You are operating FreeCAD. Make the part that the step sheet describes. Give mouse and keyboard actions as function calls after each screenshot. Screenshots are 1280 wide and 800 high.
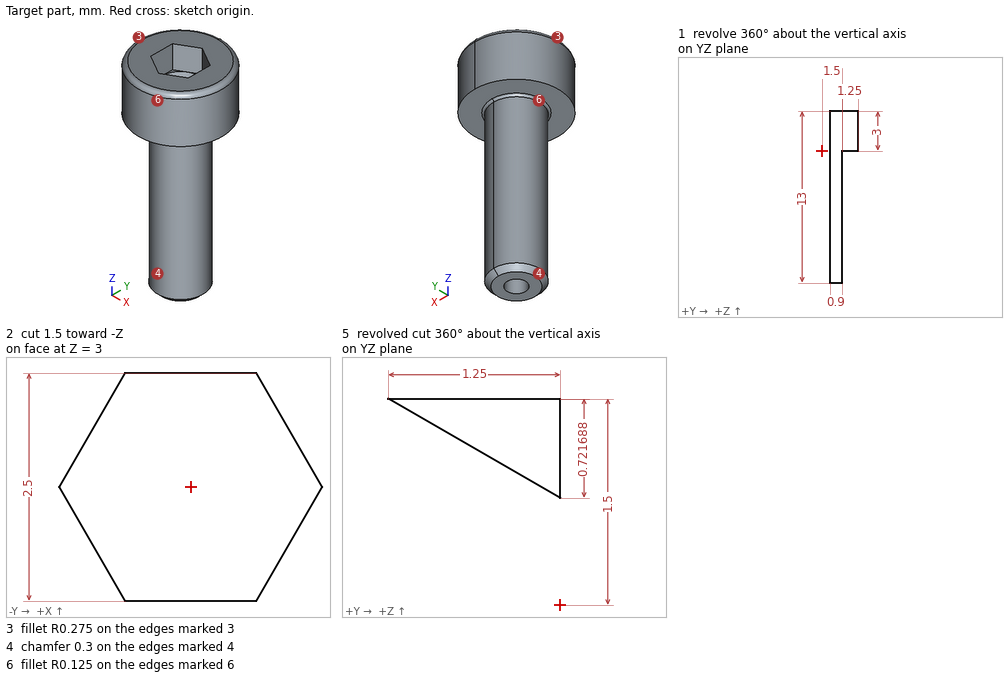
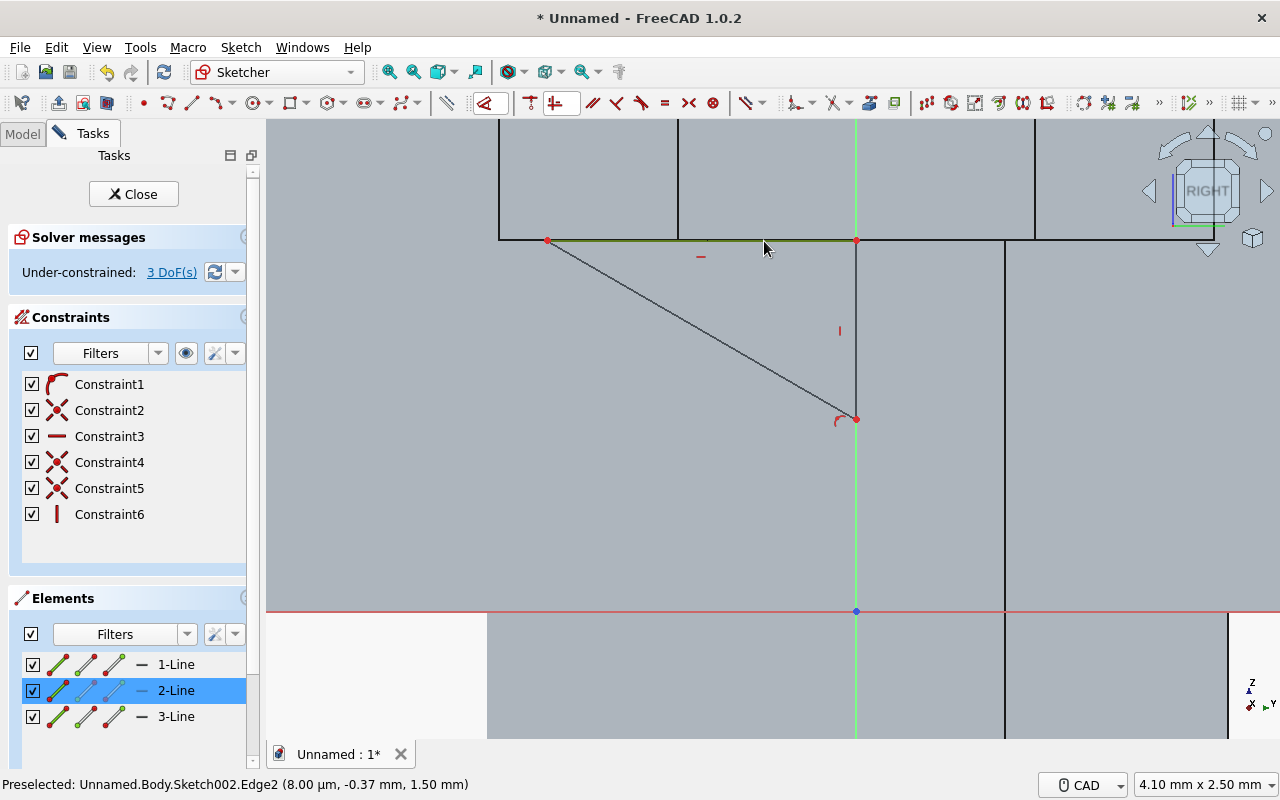
click(502, 104)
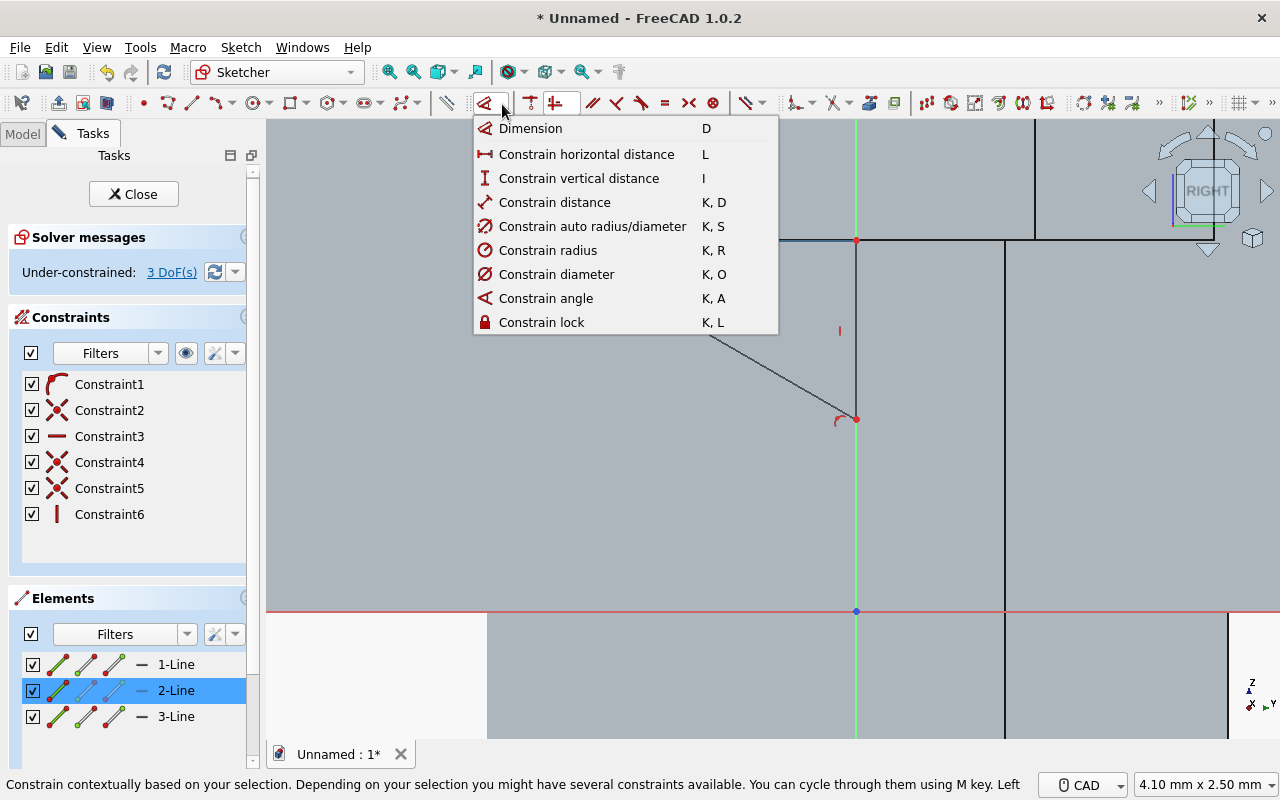
click(626, 154)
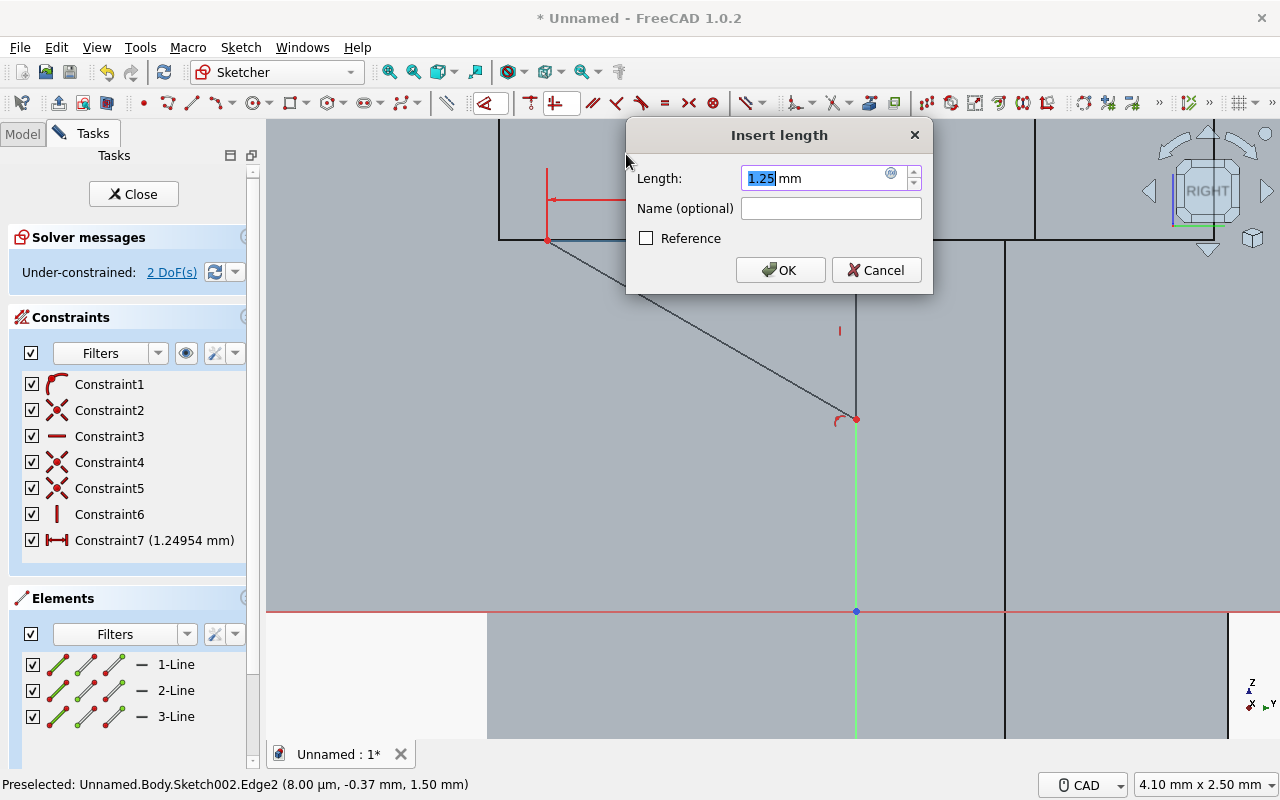
text(1.25)
key(Return)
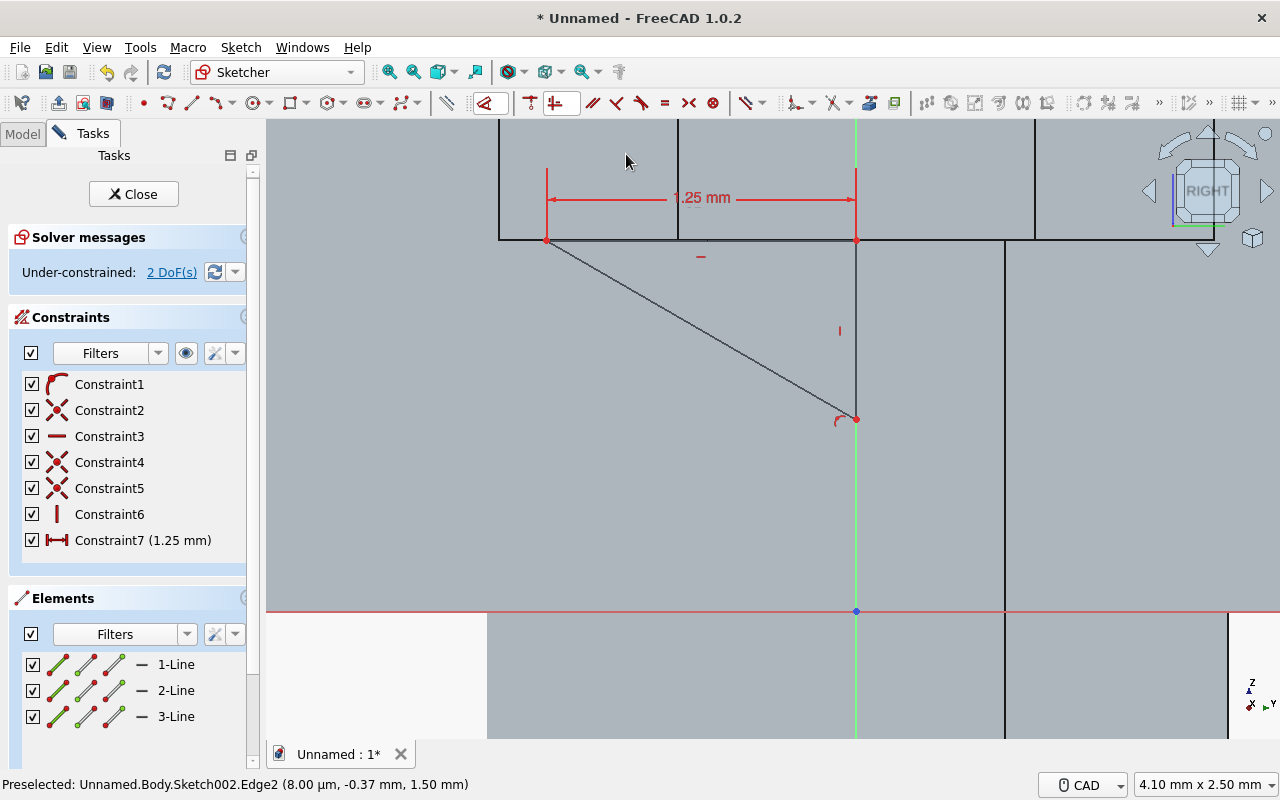
click(856, 241)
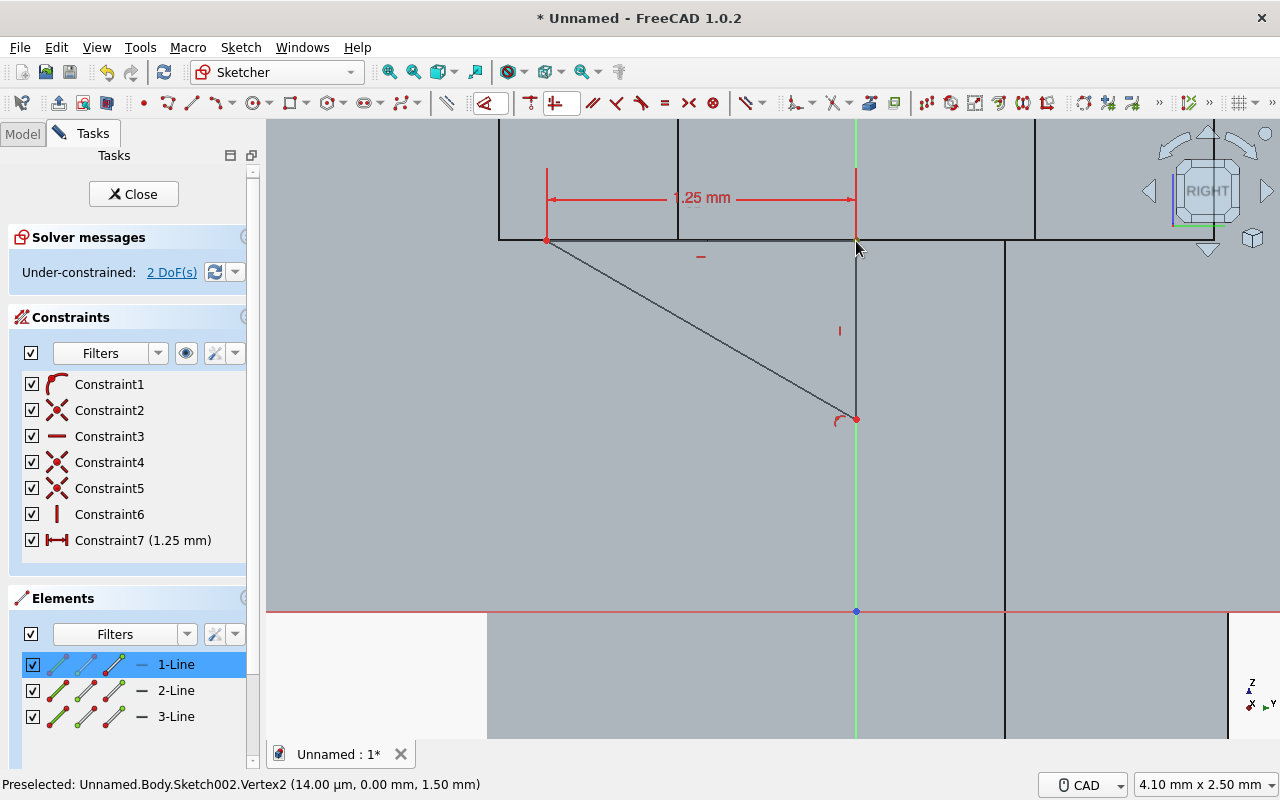
key(i)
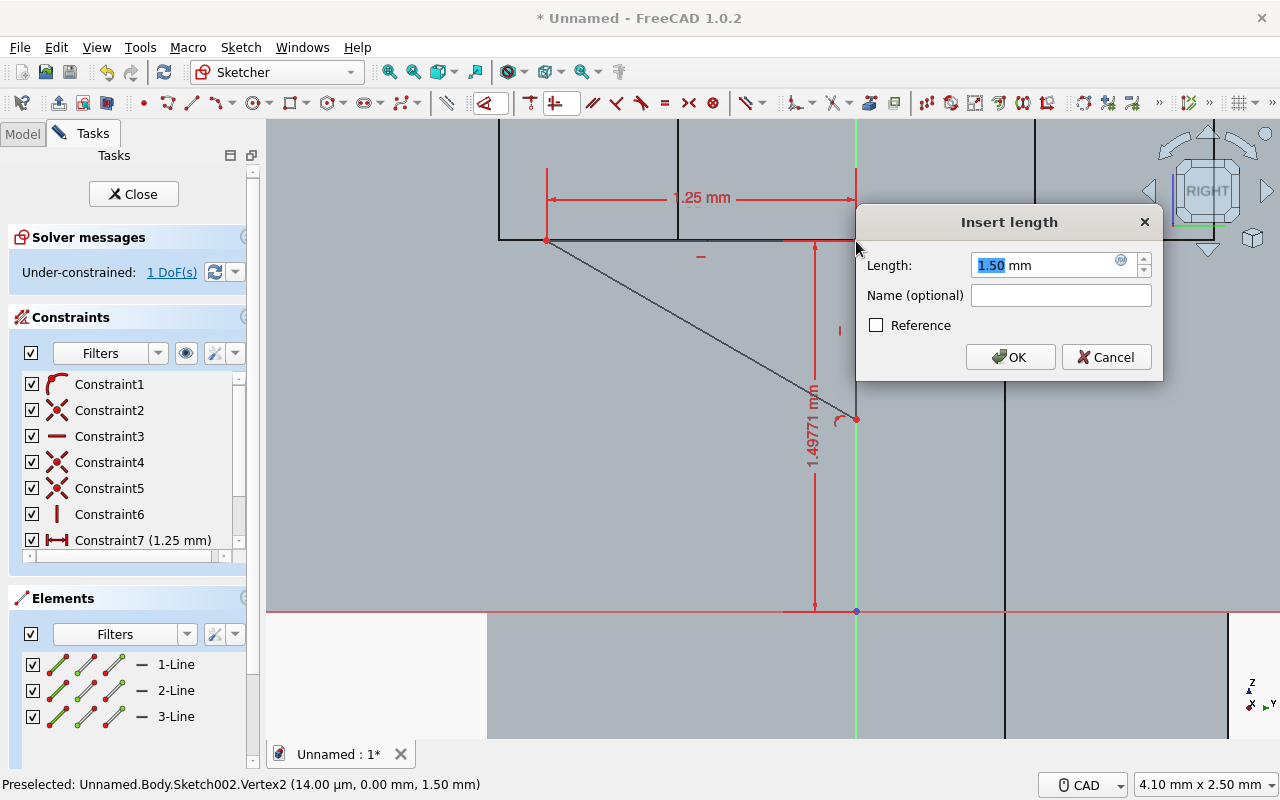
text(1.5)
key(Return)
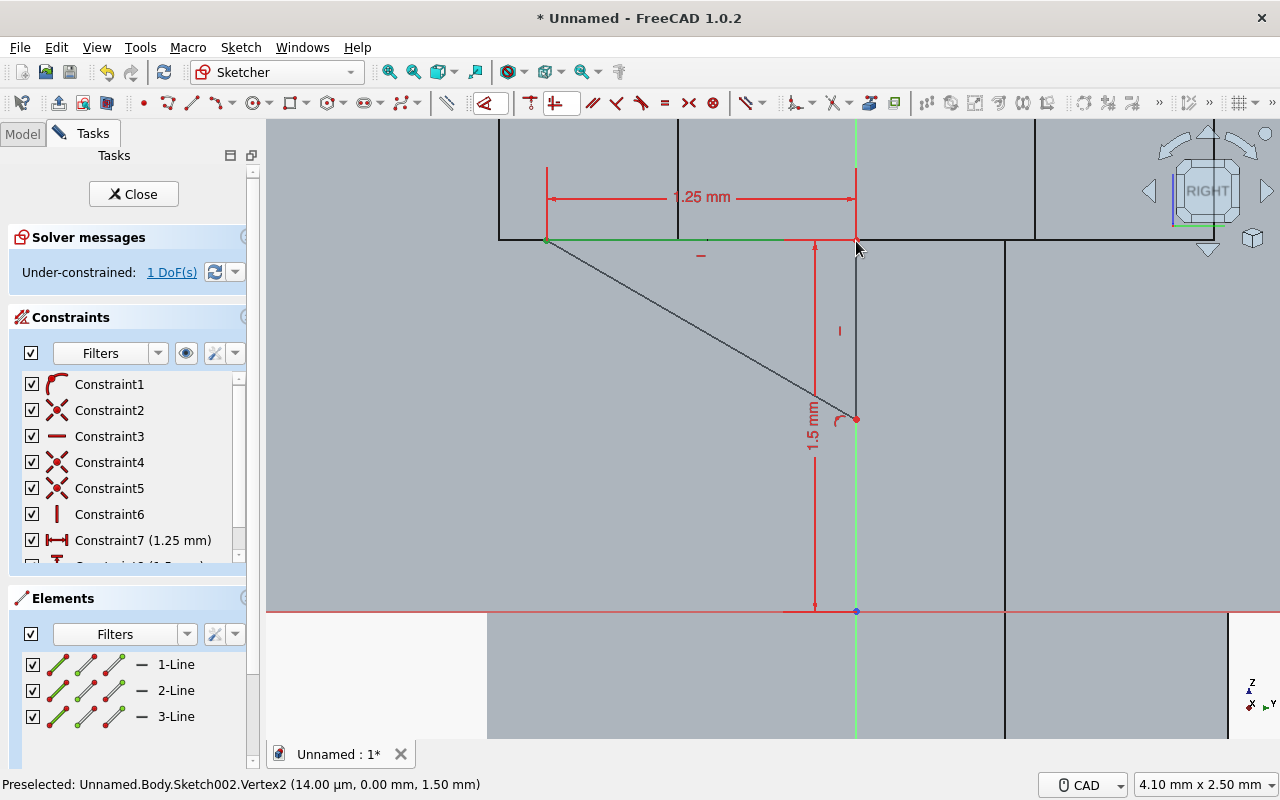
click(856, 366)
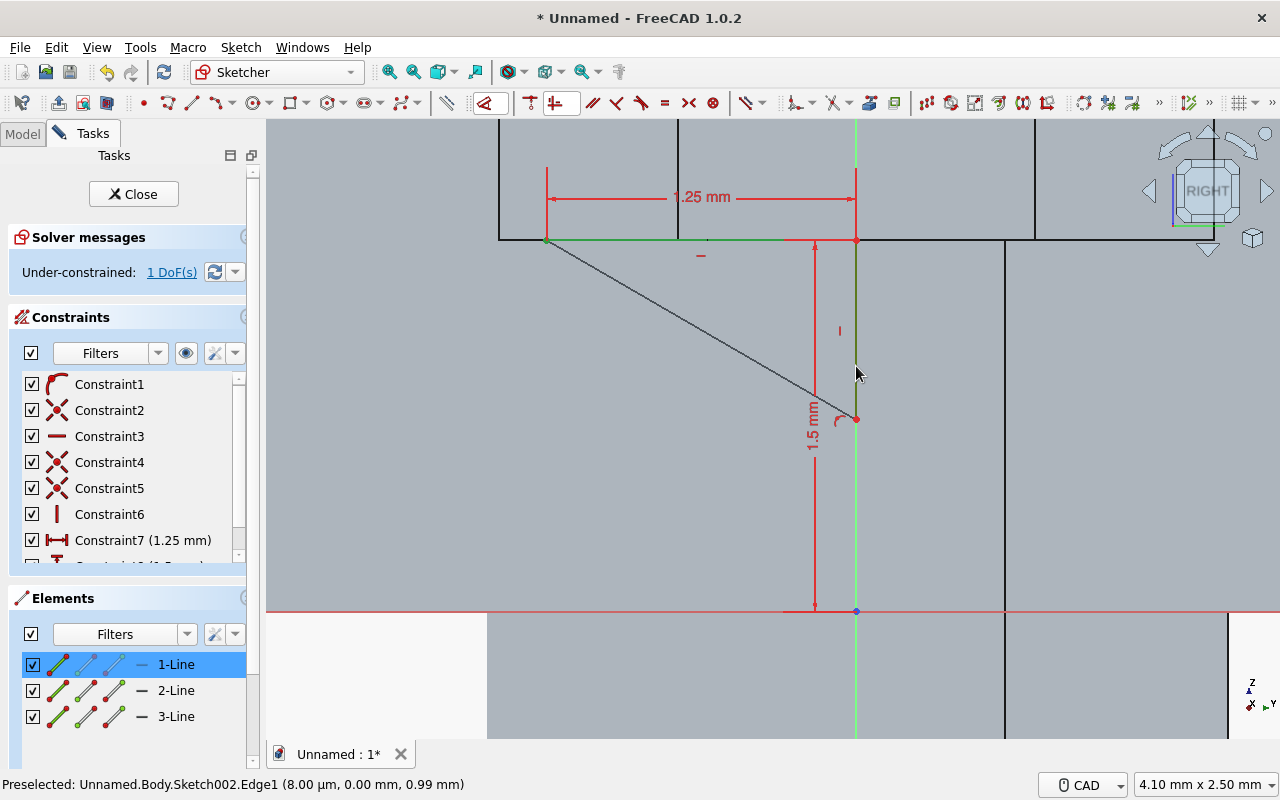
click(502, 104)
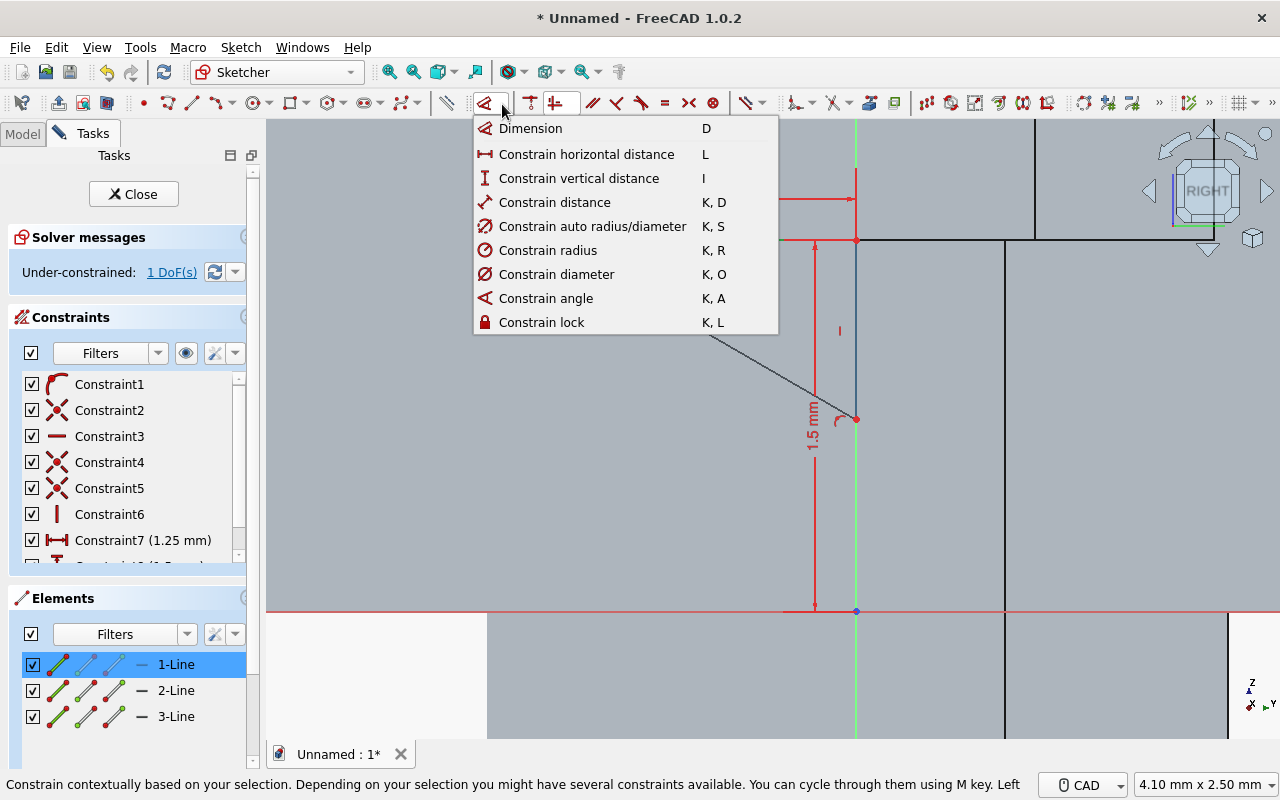
click(626, 178)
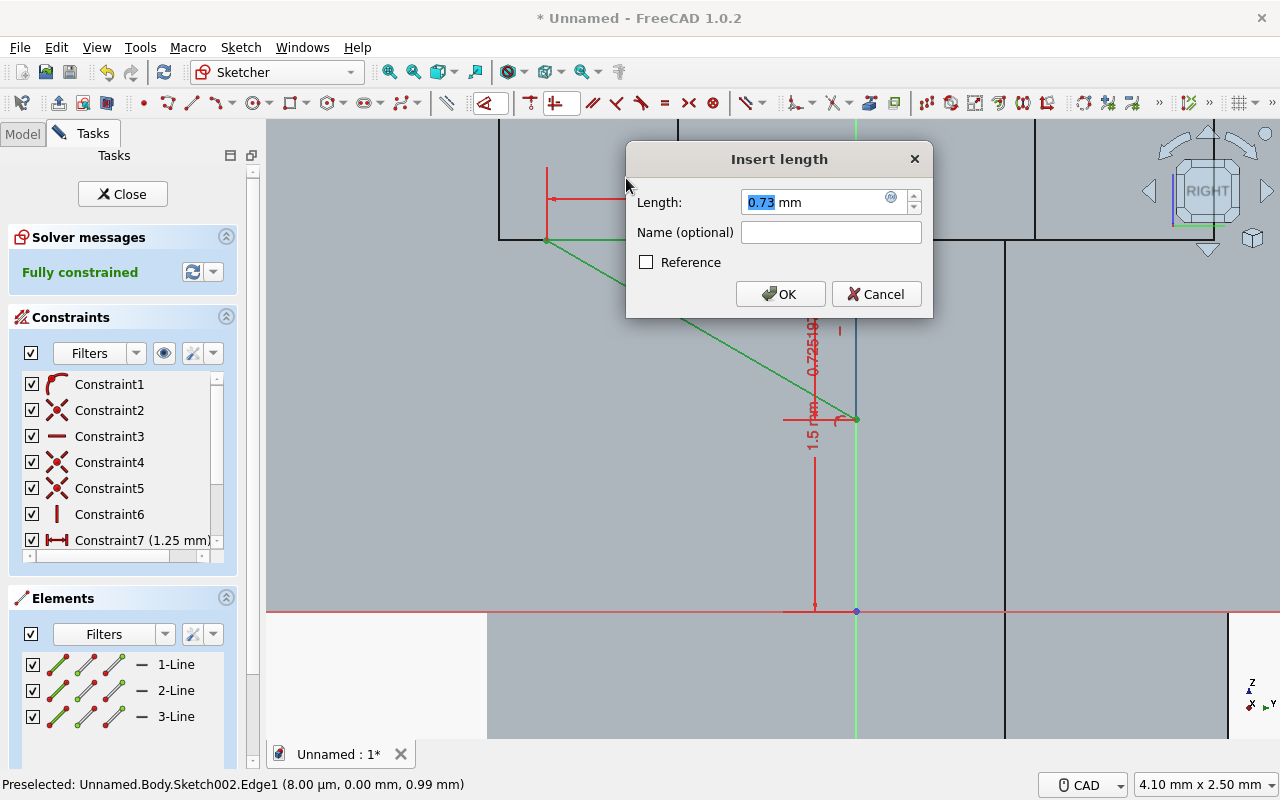
text(0.721688)
key(Return)